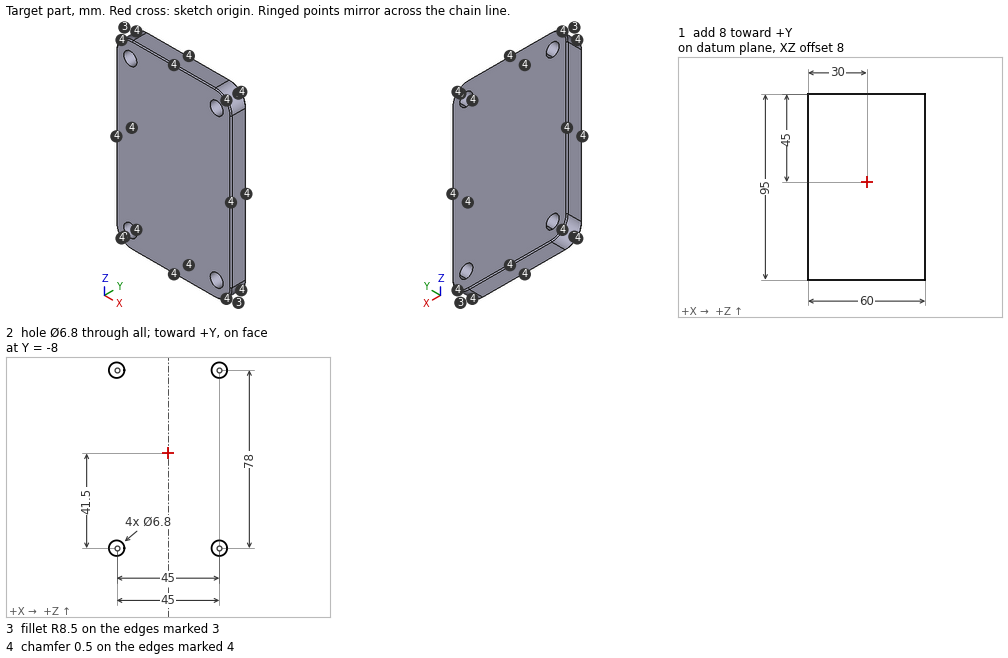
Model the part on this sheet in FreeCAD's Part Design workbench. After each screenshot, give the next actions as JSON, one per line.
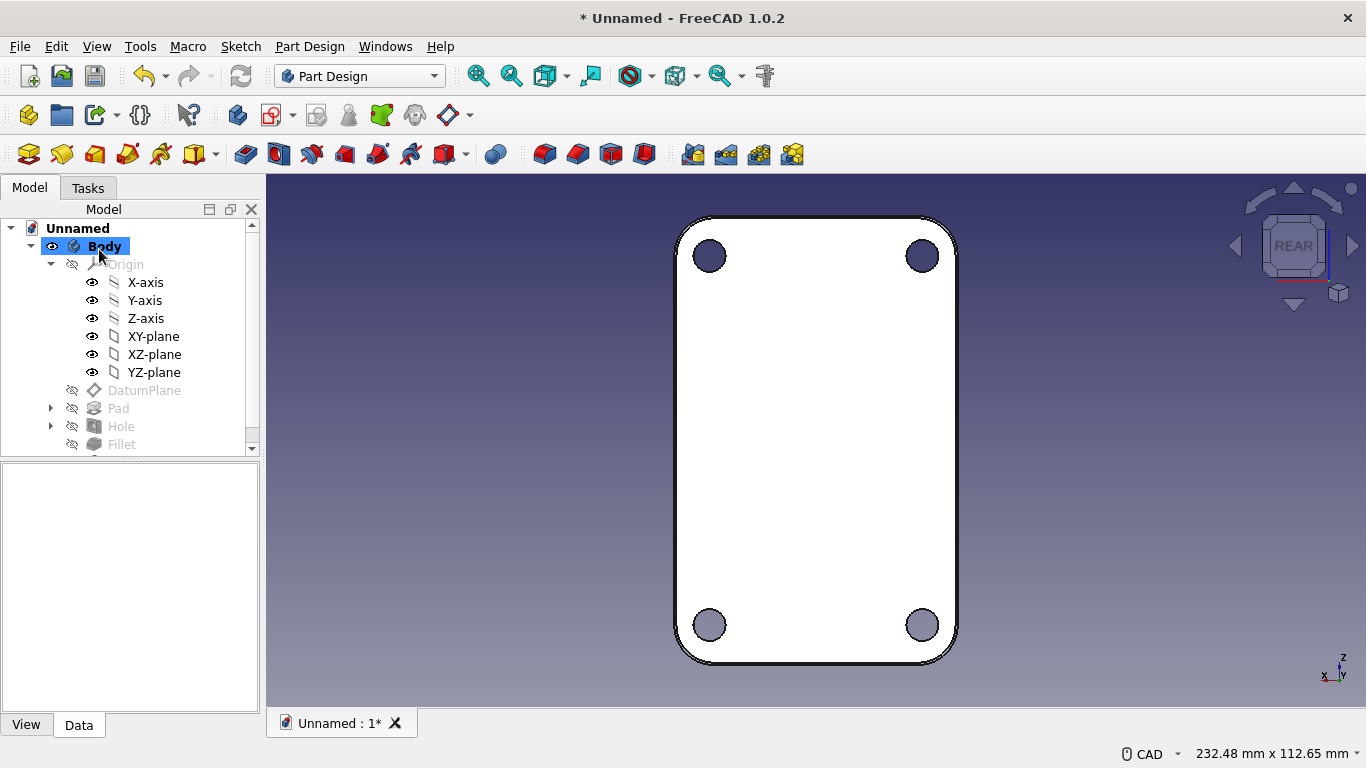
{"action": "key", "text": "0"}